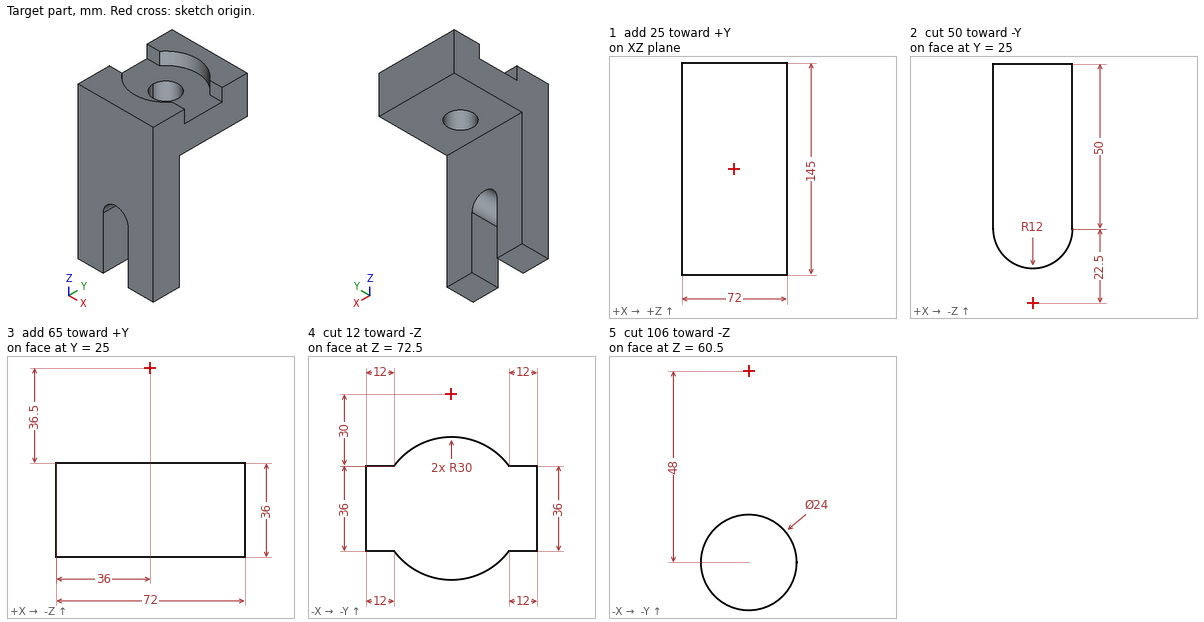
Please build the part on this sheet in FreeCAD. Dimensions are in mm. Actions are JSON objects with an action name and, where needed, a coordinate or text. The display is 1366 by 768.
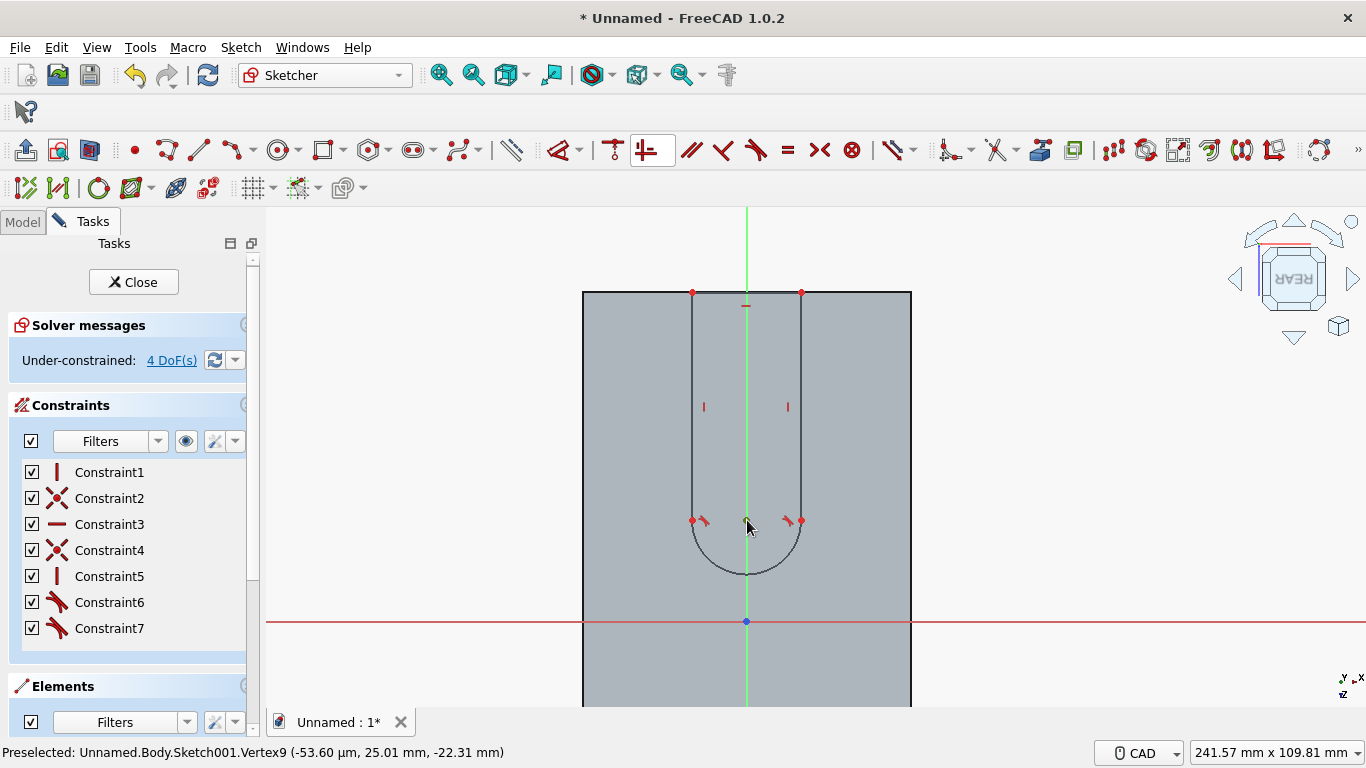
{"action": "left_click", "coordinate": [747, 489]}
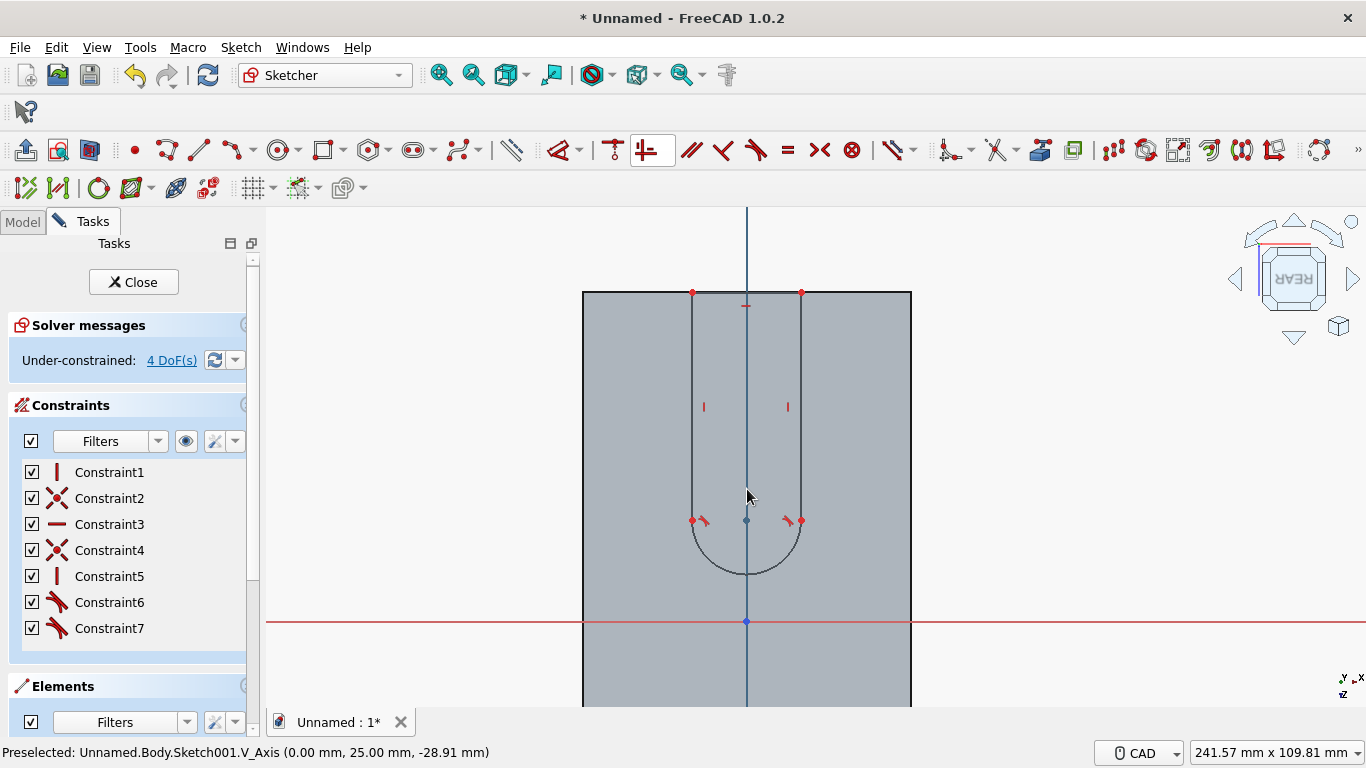
{"action": "left_click", "coordinate": [614, 150]}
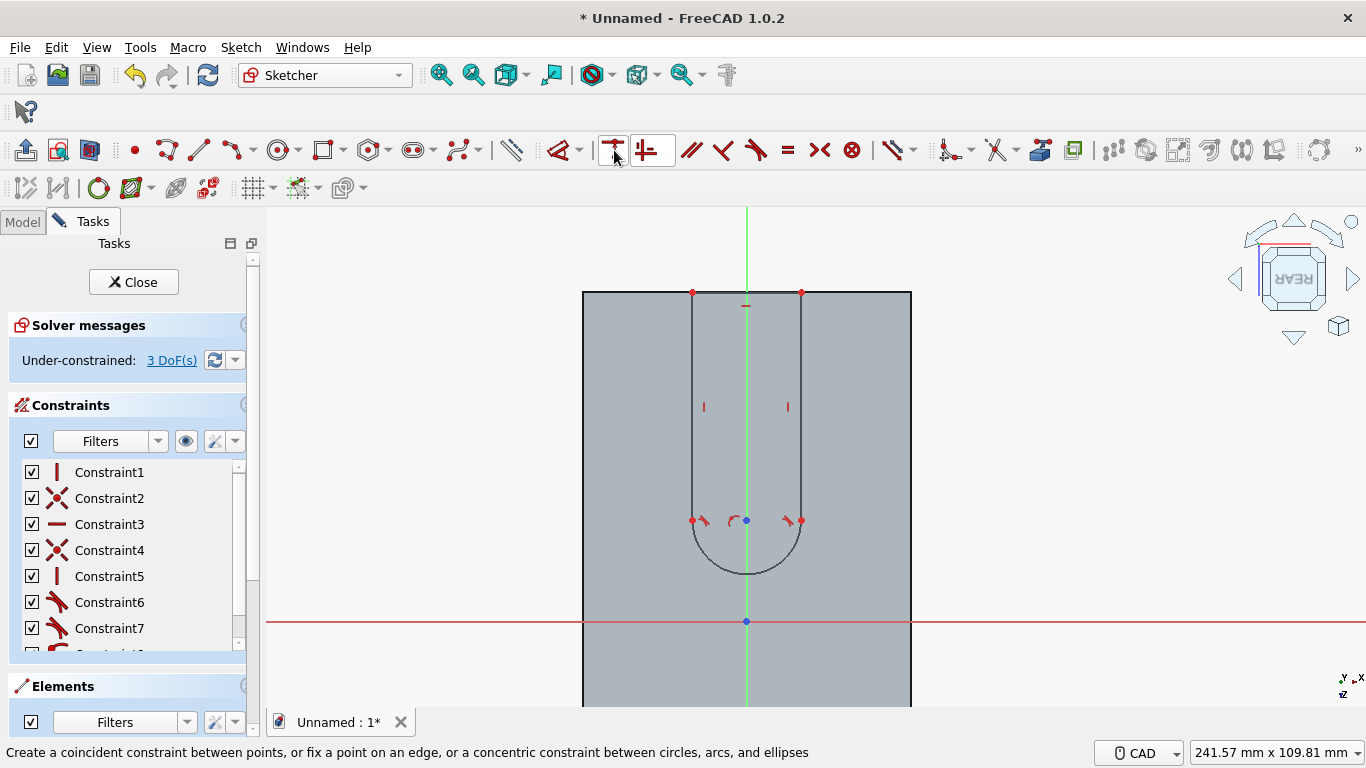
{"action": "left_click", "coordinate": [558, 150]}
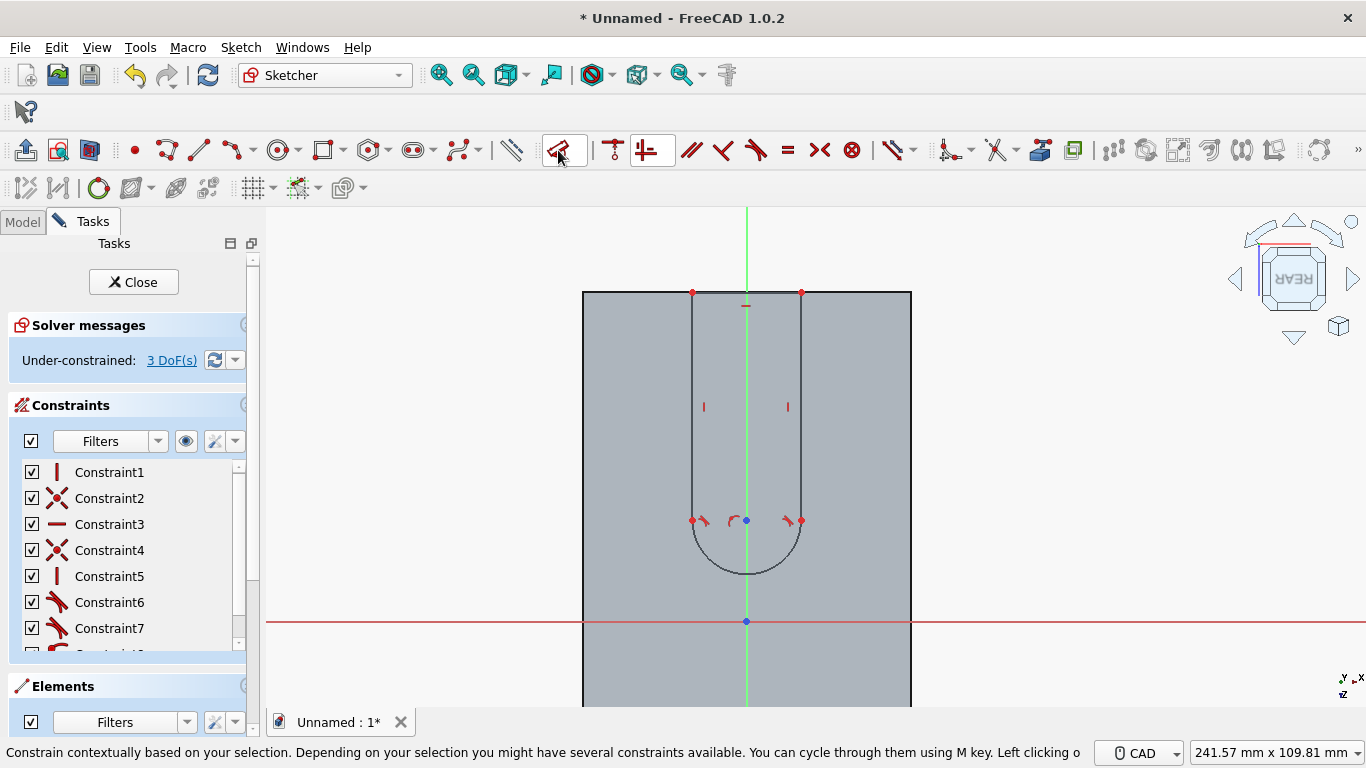
{"action": "left_click", "coordinate": [715, 564]}
{"action": "left_click", "coordinate": [696, 590]}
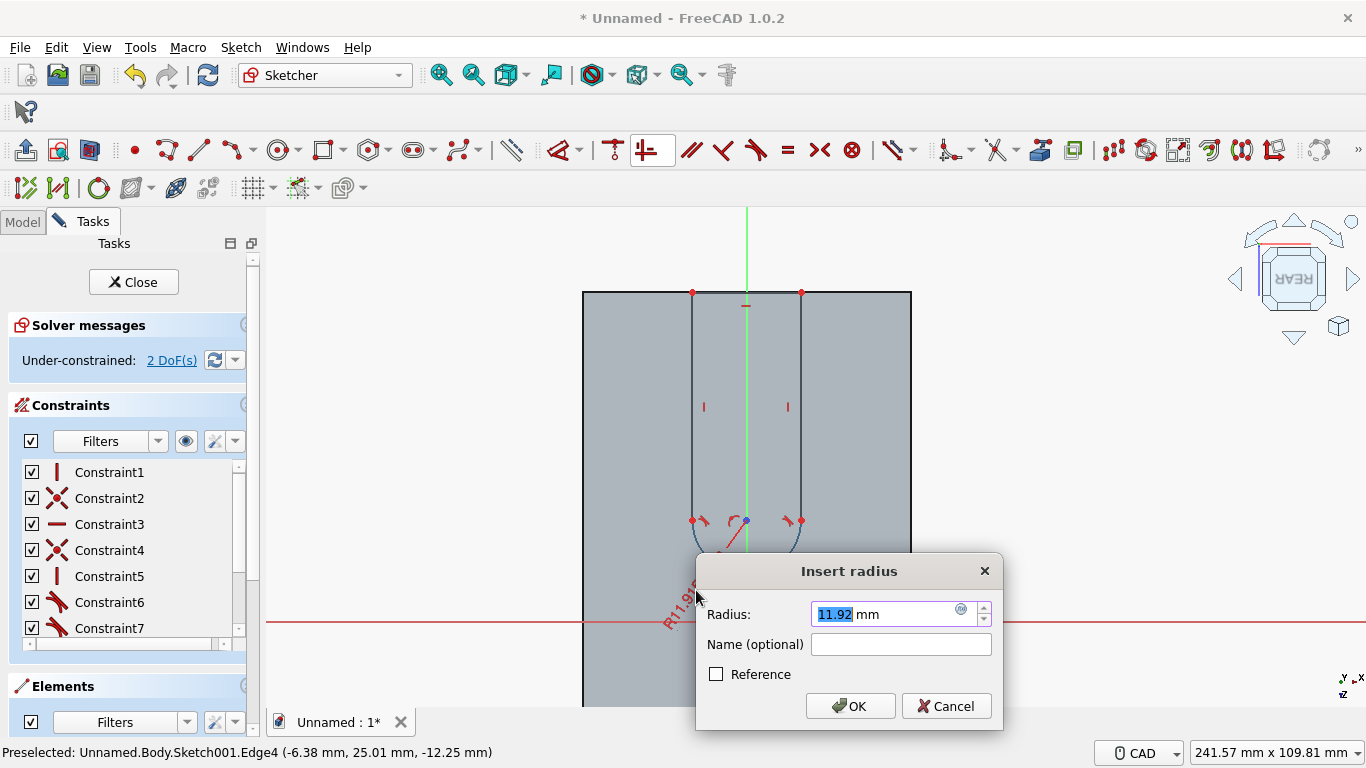
{"action": "type", "text": "12"}
{"action": "key", "text": "Return"}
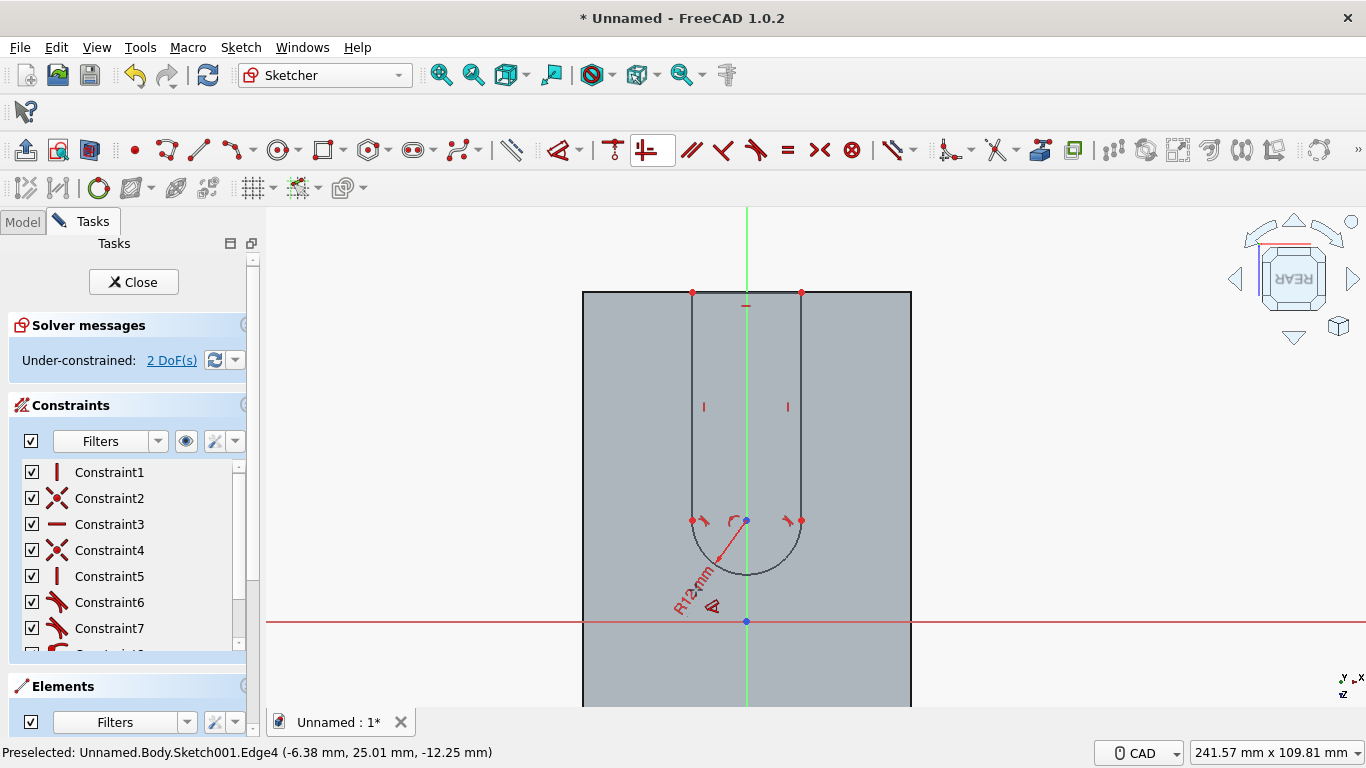
{"action": "left_click", "coordinate": [801, 452]}
{"action": "left_click", "coordinate": [835, 407]}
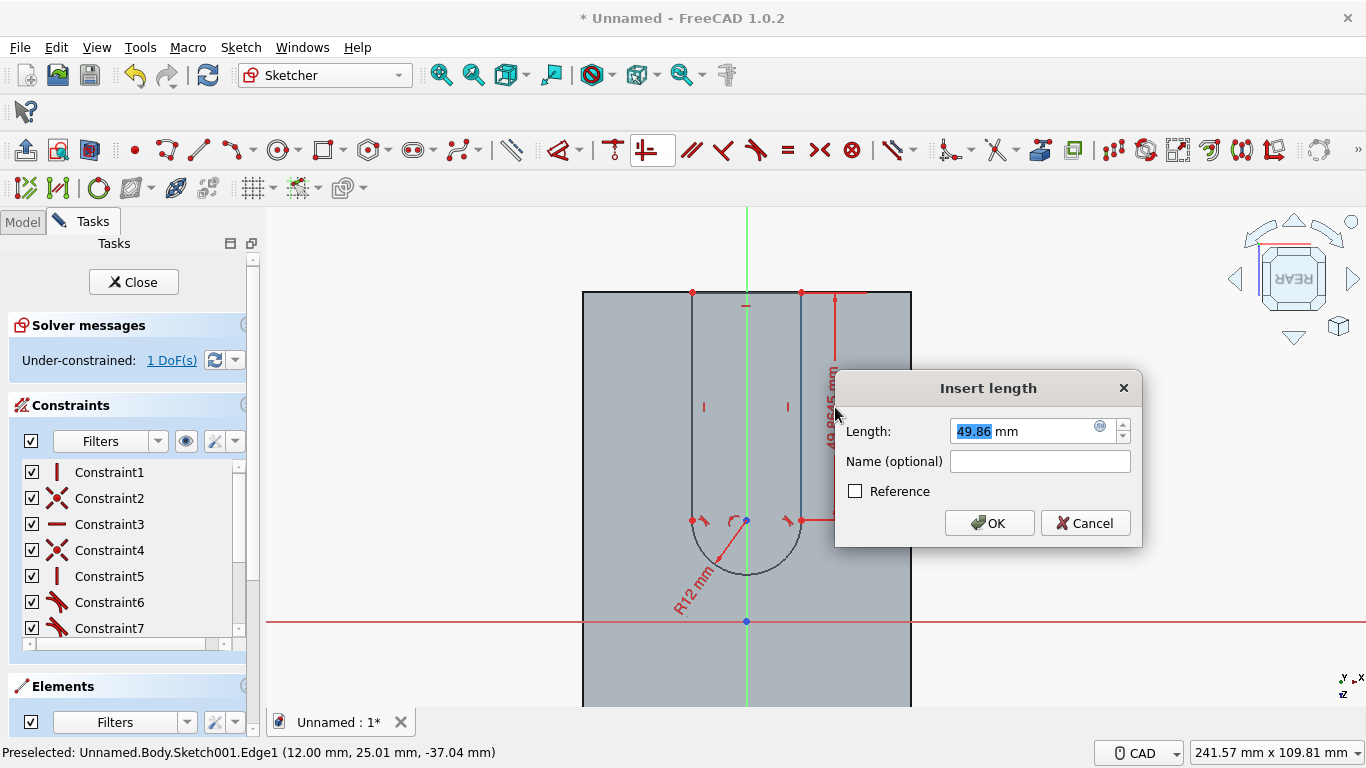
{"action": "type", "text": "50"}
{"action": "key", "text": "Return"}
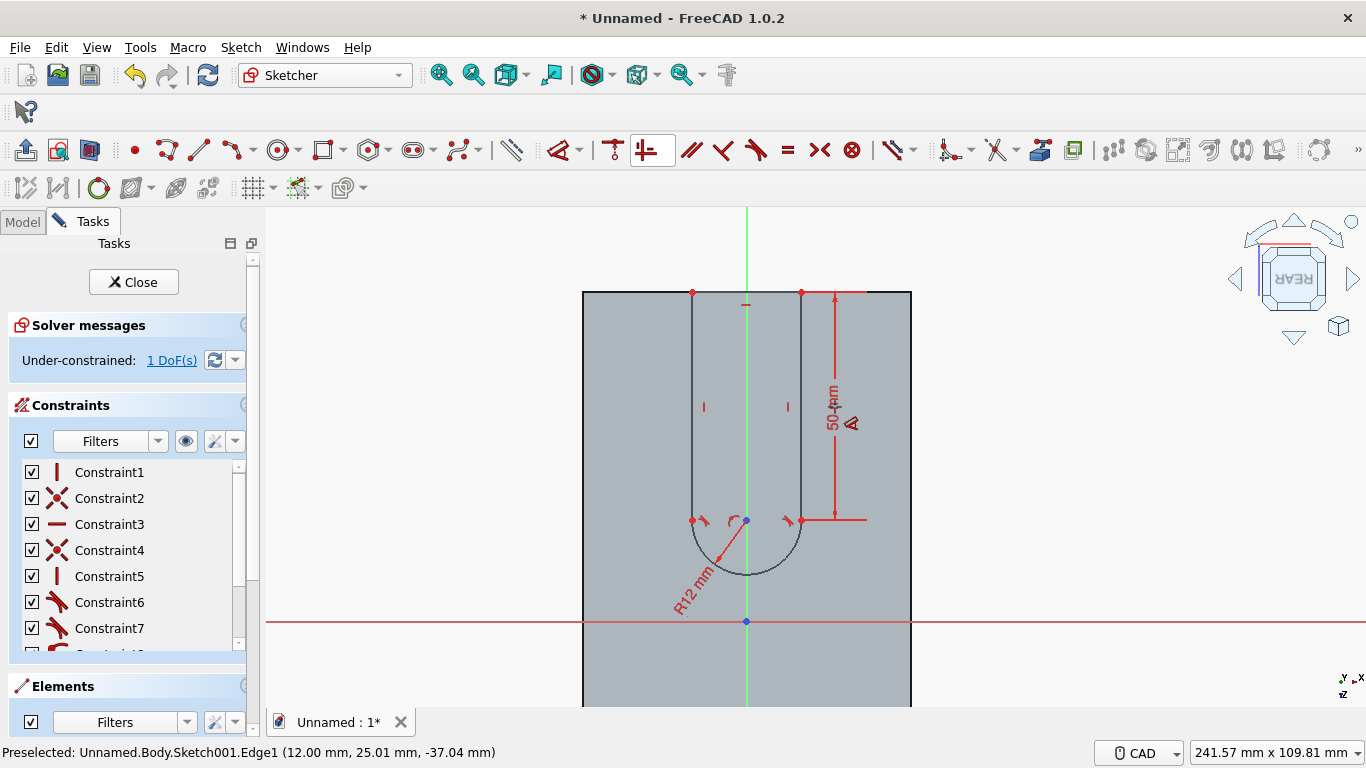
{"action": "left_click", "coordinate": [801, 520]}
{"action": "left_click", "coordinate": [835, 571]}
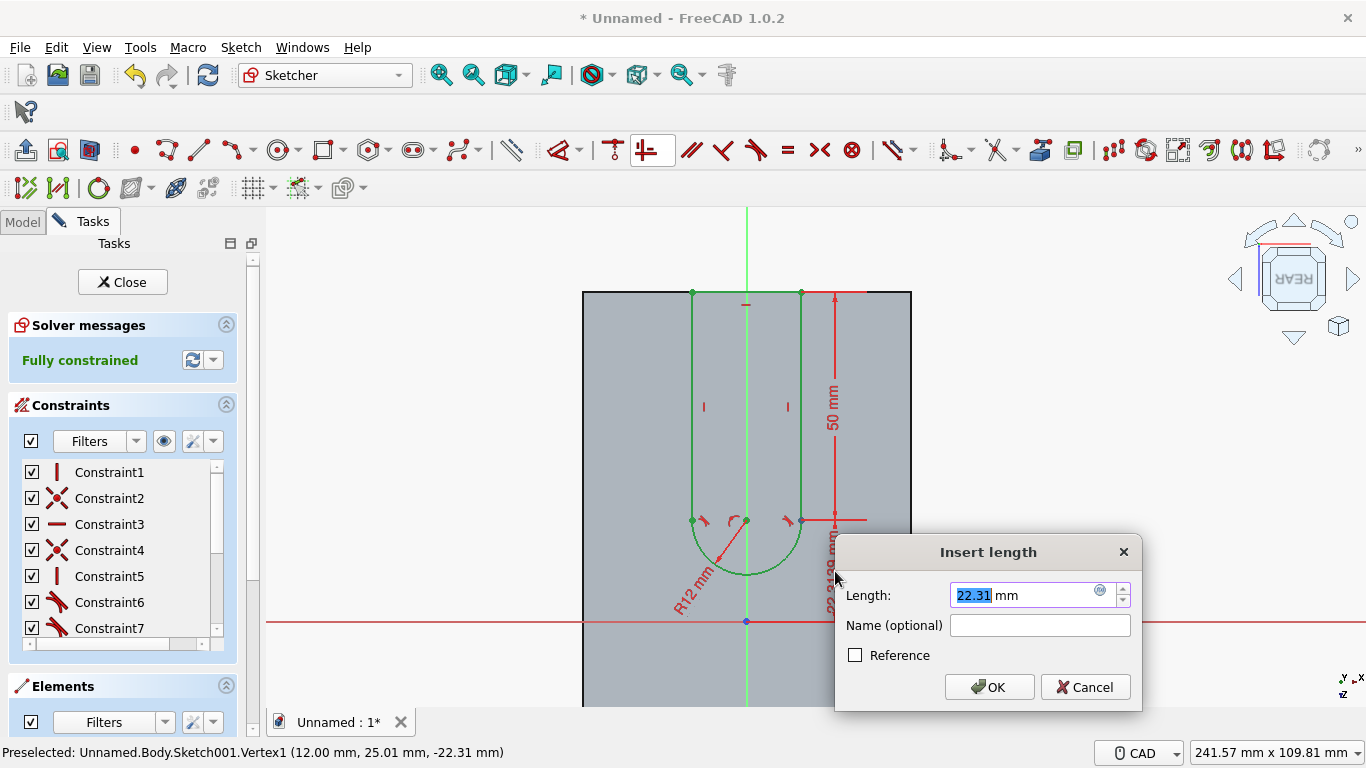
{"action": "type", "text": "22.5"}
{"action": "key", "text": "Return"}
{"action": "key", "text": "Escape"}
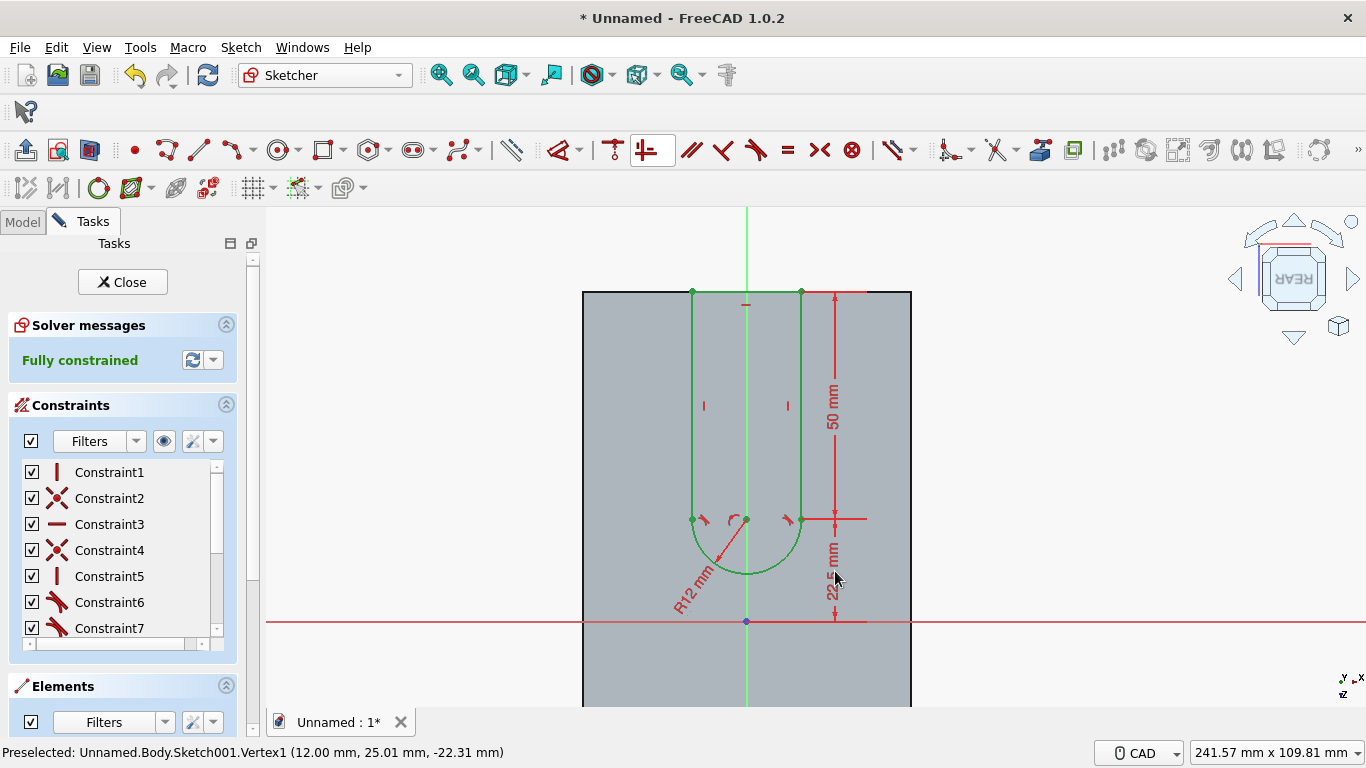
{"action": "left_click", "coordinate": [123, 282]}